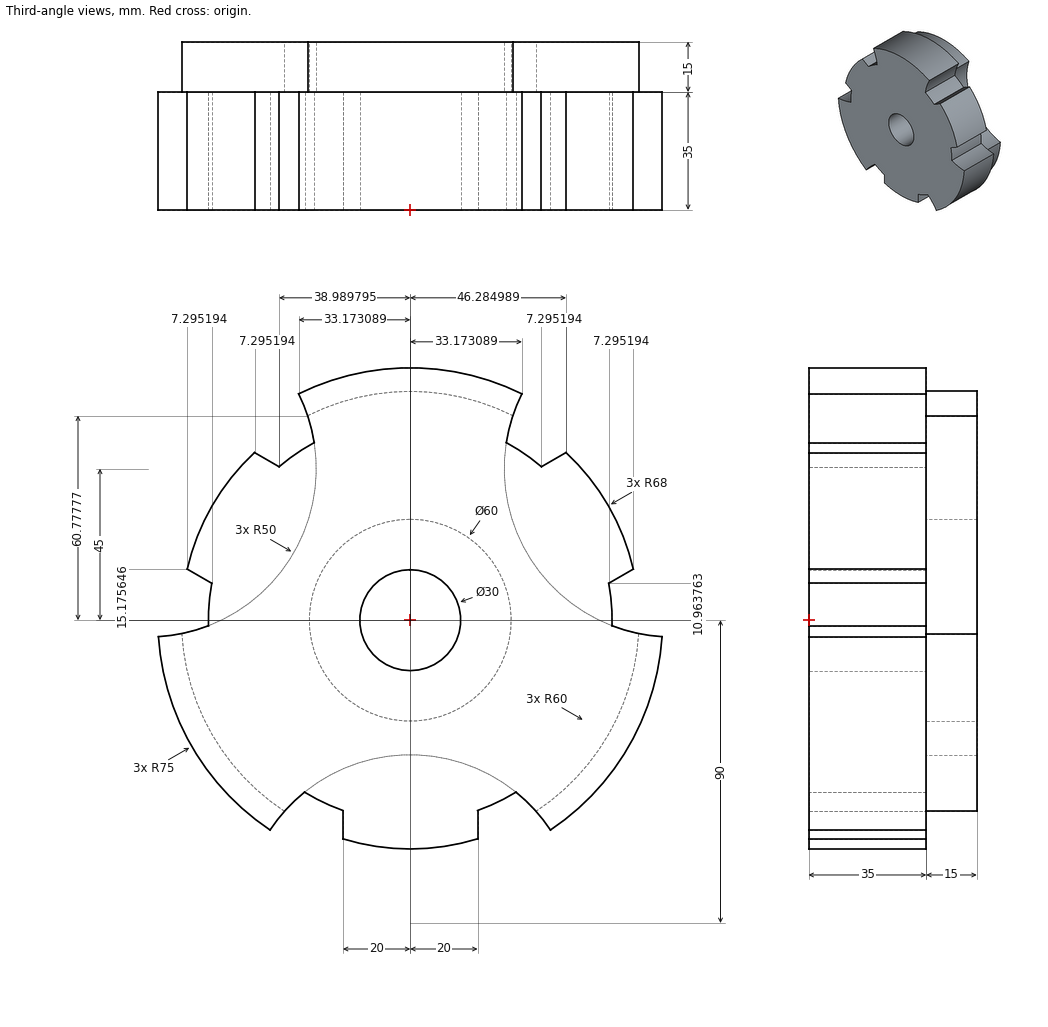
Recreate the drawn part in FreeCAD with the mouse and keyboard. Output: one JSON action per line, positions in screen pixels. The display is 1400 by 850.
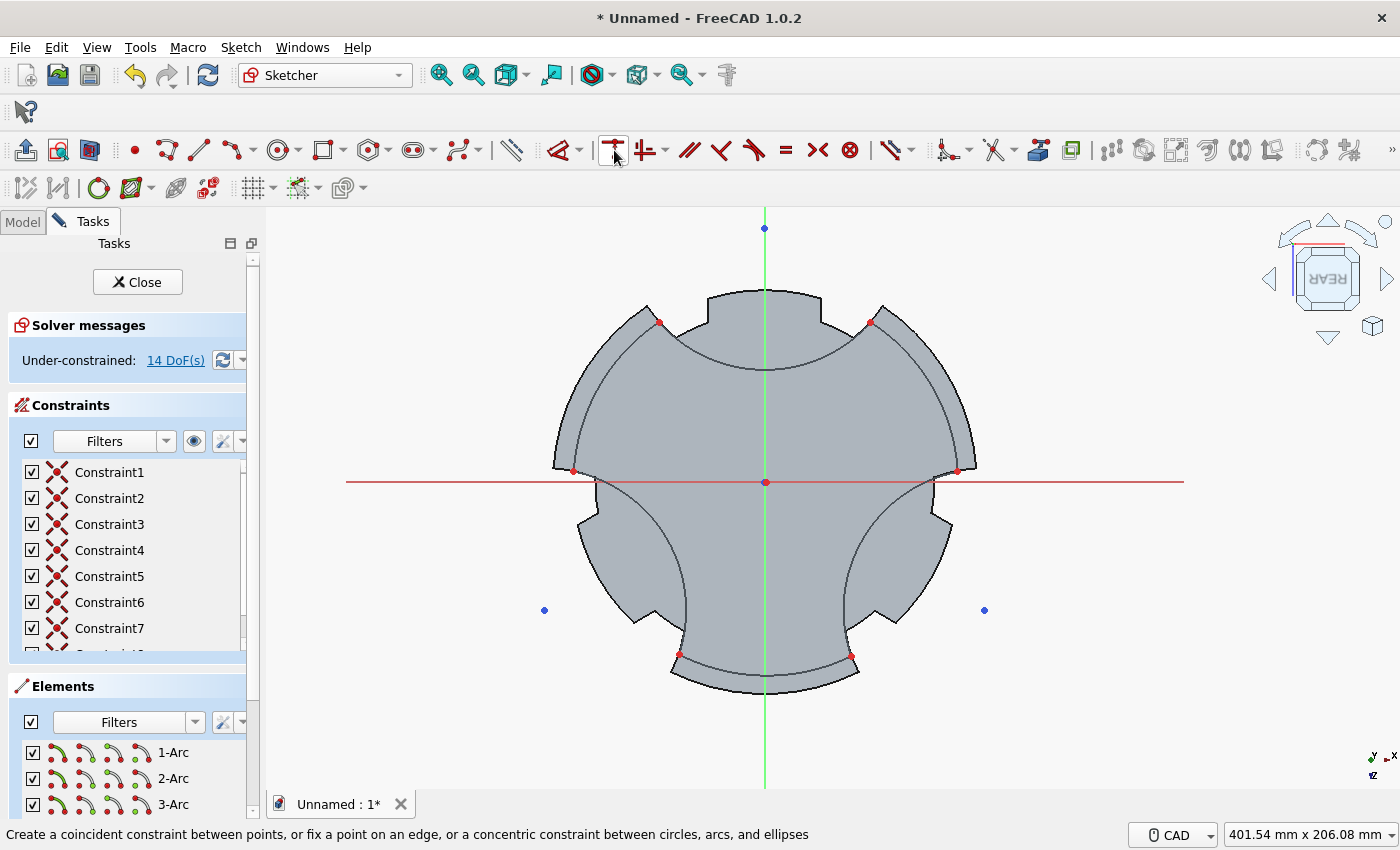
{"action": "left_click_drag", "start_coordinate": [755, 472], "coordinate": [777, 493]}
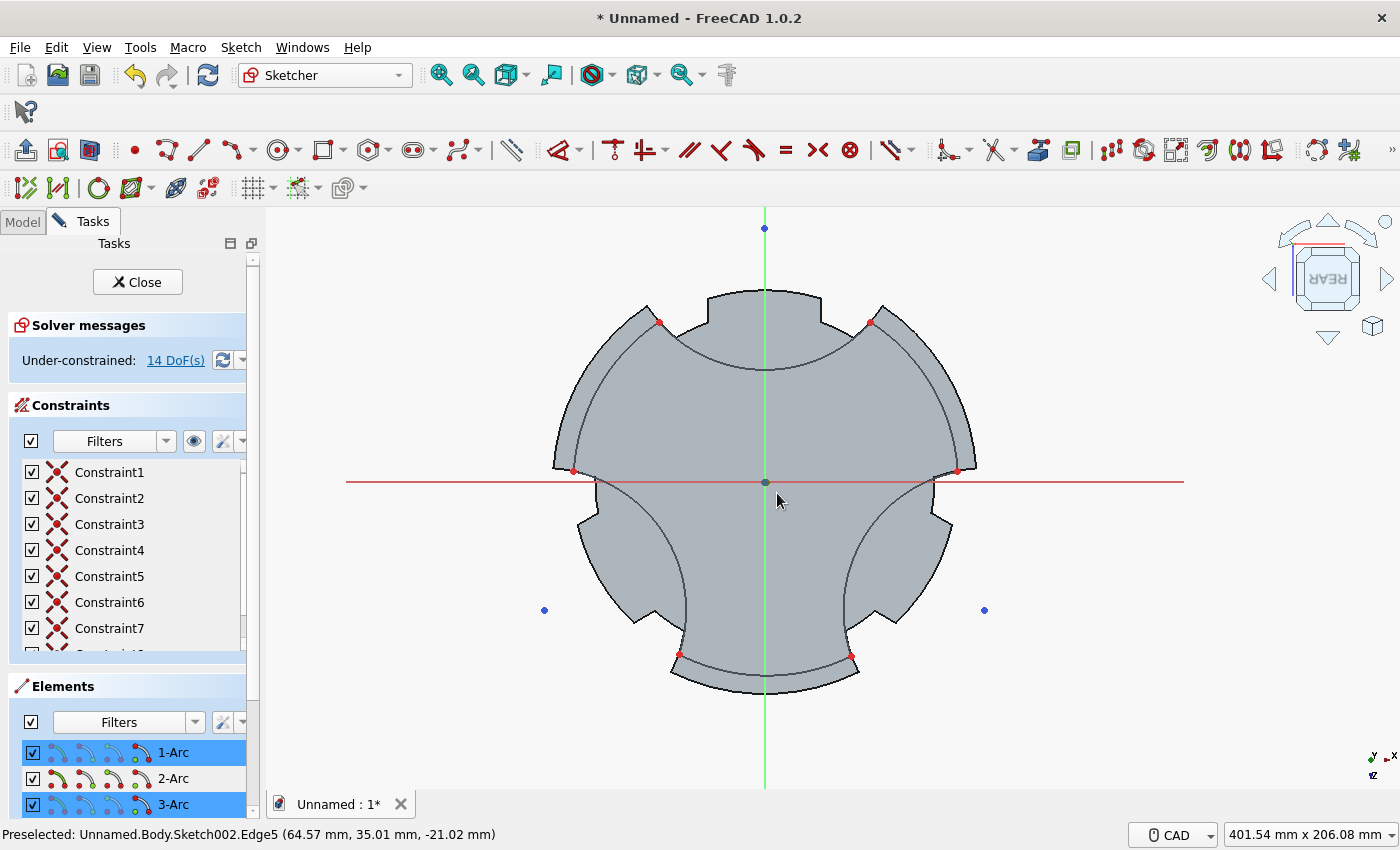
{"action": "left_click", "coordinate": [614, 150]}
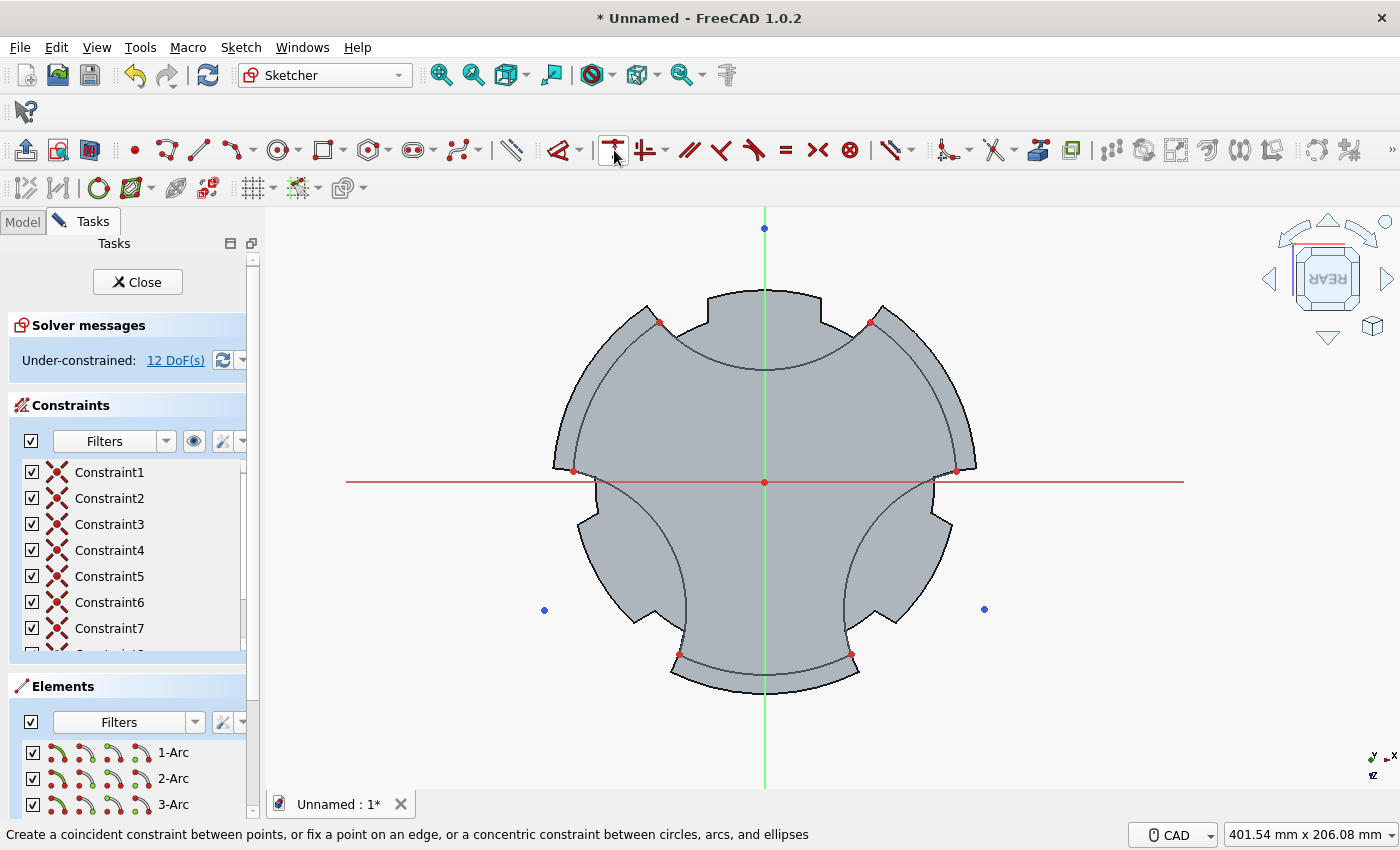
{"action": "left_click", "coordinate": [619, 358]}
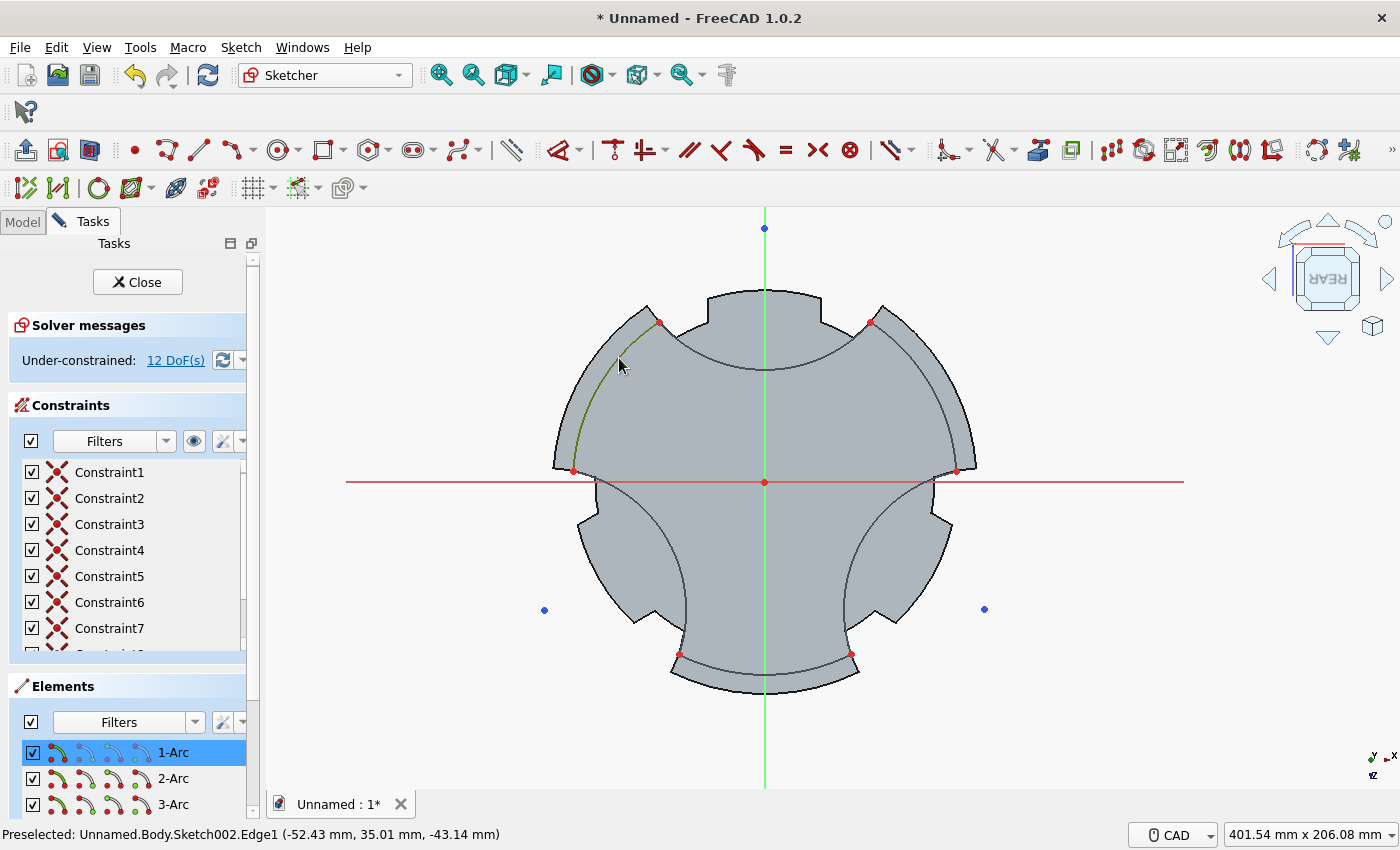
{"action": "left_click", "coordinate": [730, 672]}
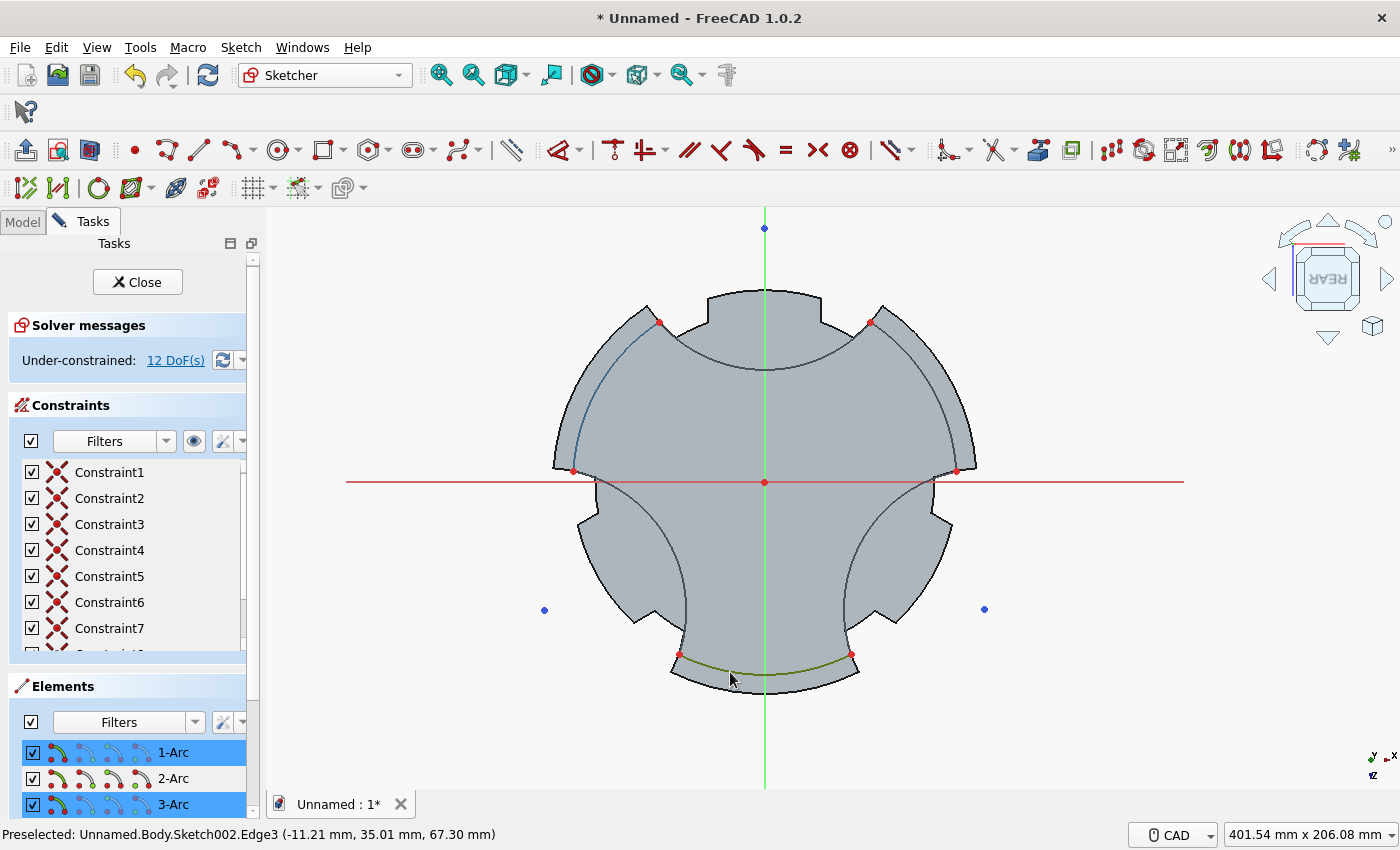
{"action": "left_click", "coordinate": [946, 419]}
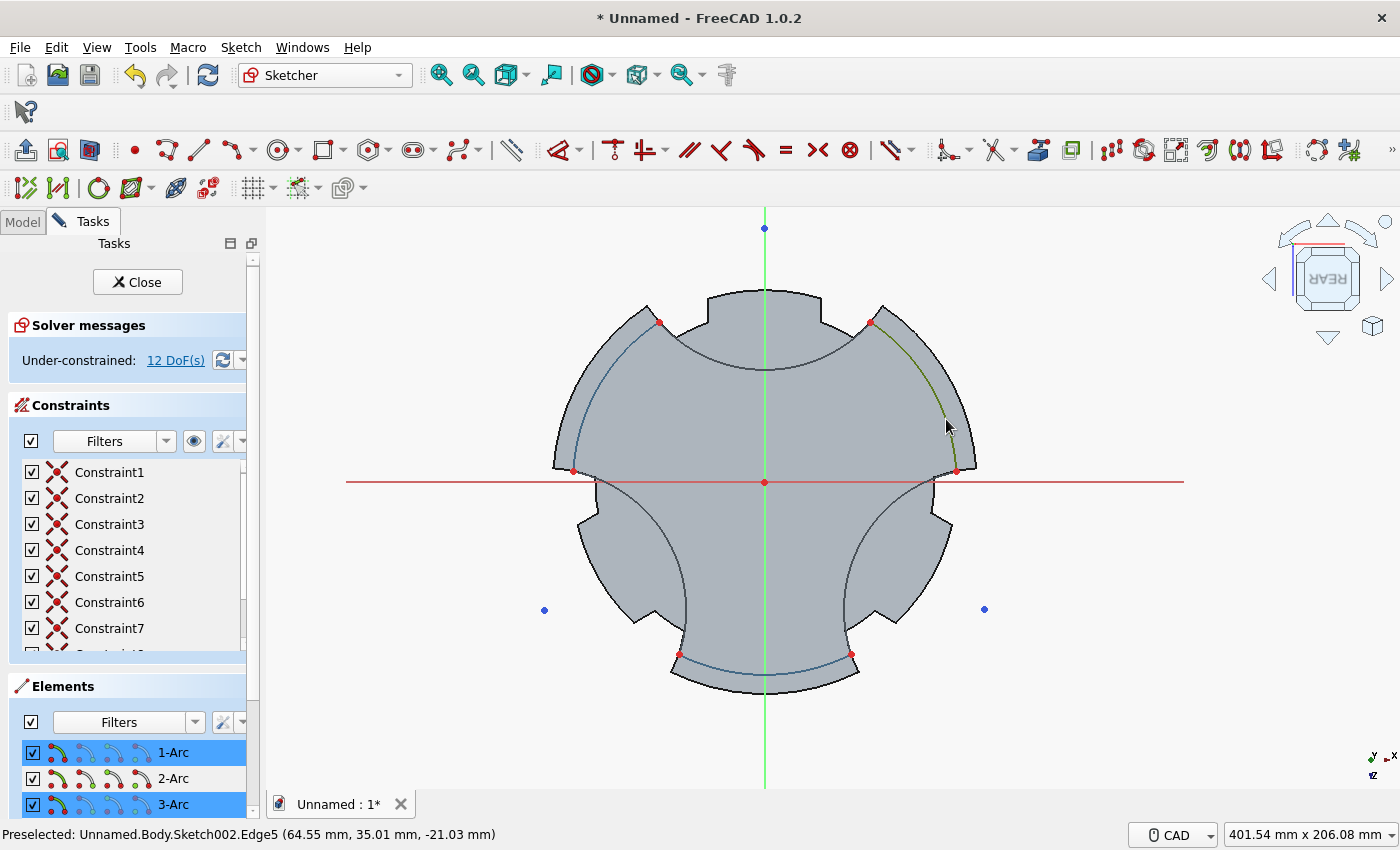
{"action": "left_click", "coordinate": [786, 150]}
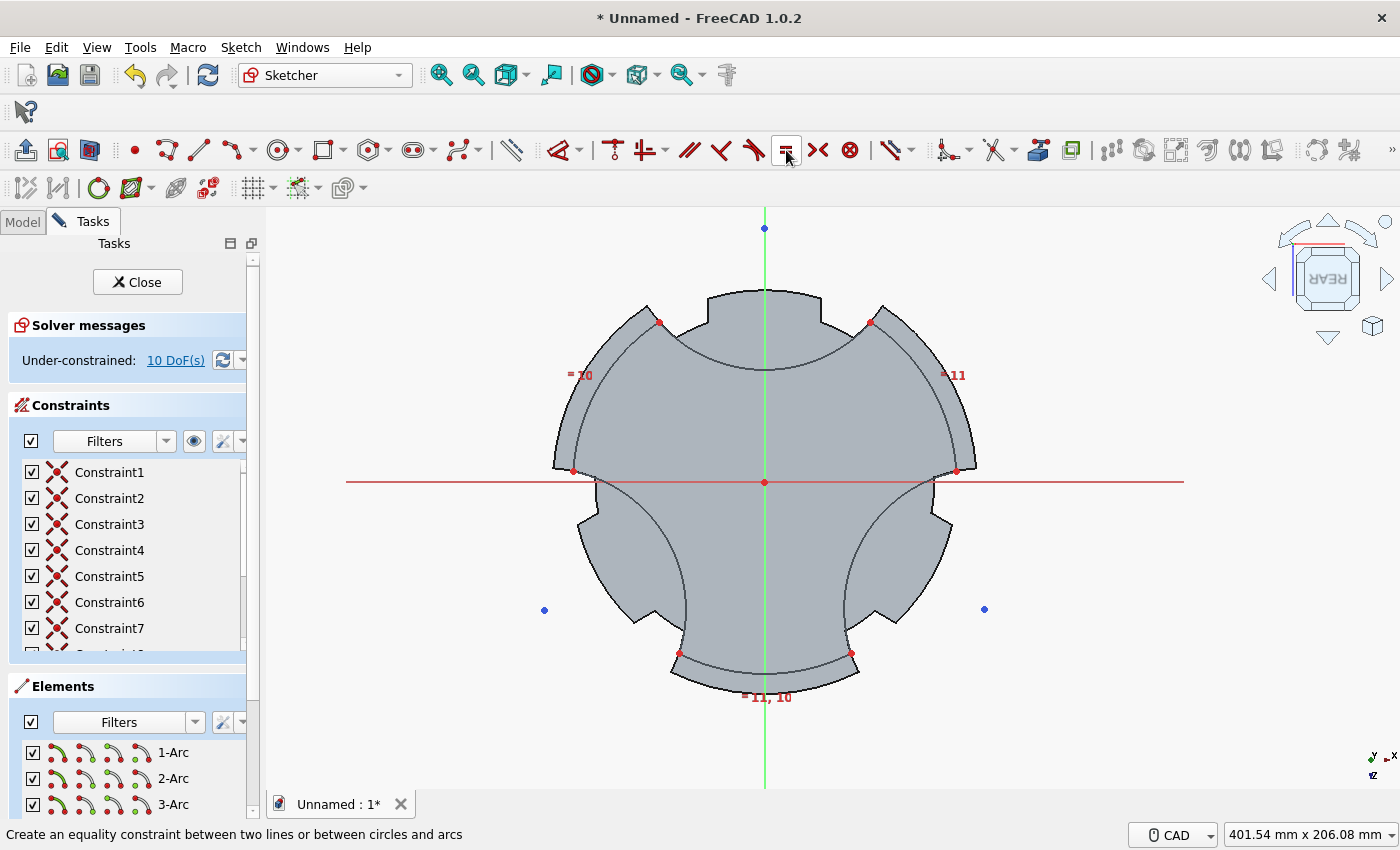
{"action": "left_click", "coordinate": [683, 583]}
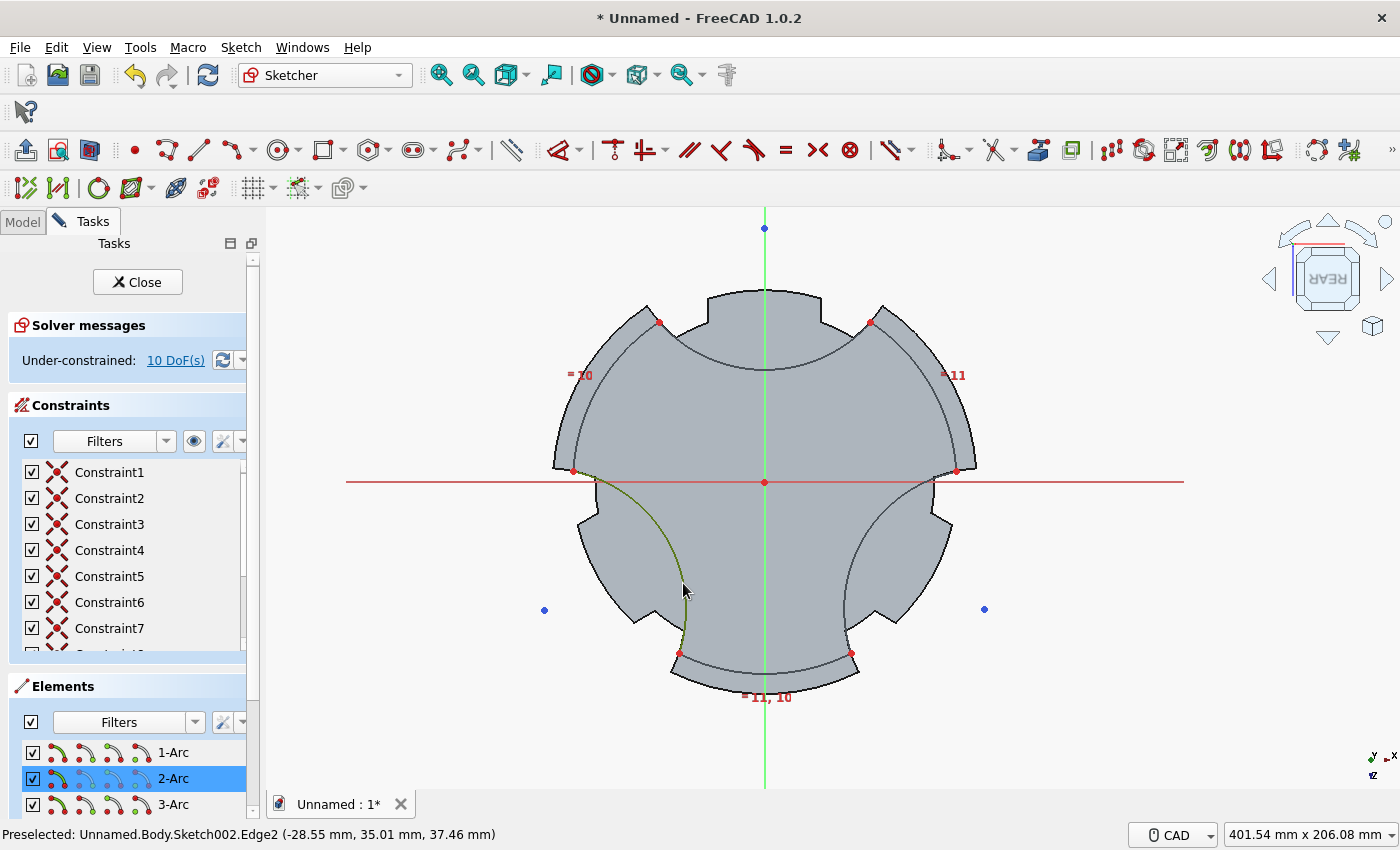
{"action": "left_click", "coordinate": [893, 503]}